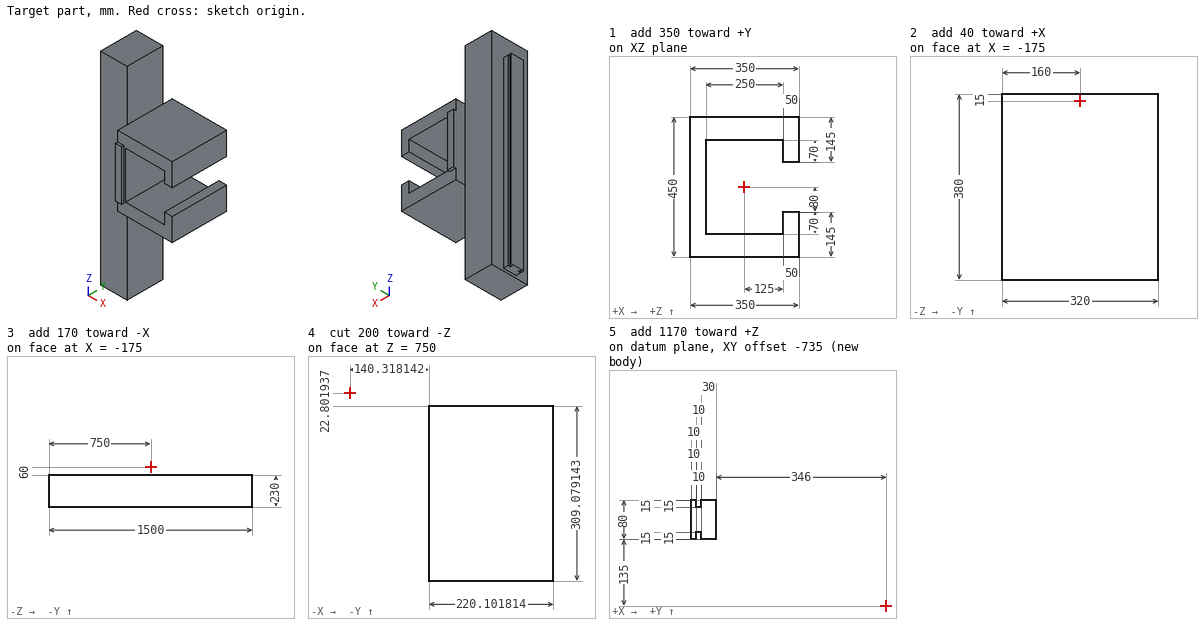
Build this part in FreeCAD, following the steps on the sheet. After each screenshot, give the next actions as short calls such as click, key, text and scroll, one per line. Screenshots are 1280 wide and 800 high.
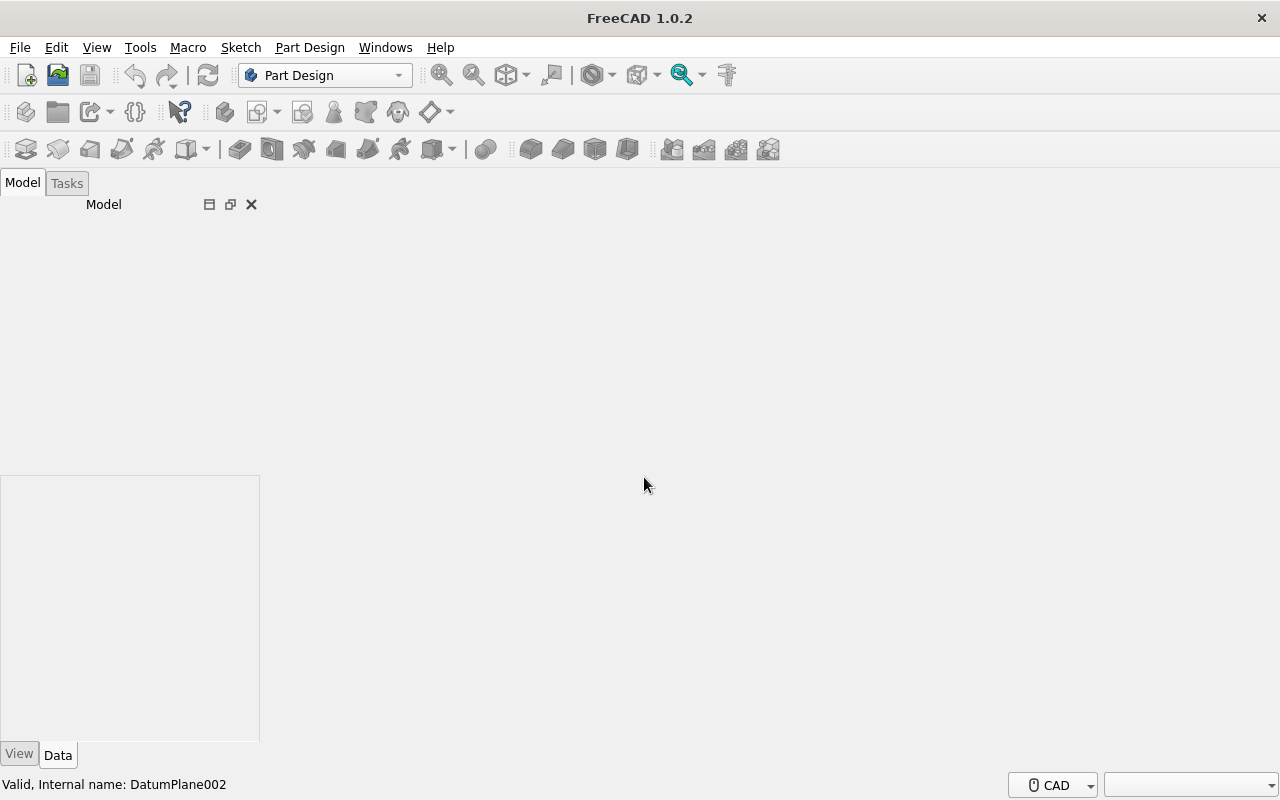
click(26, 76)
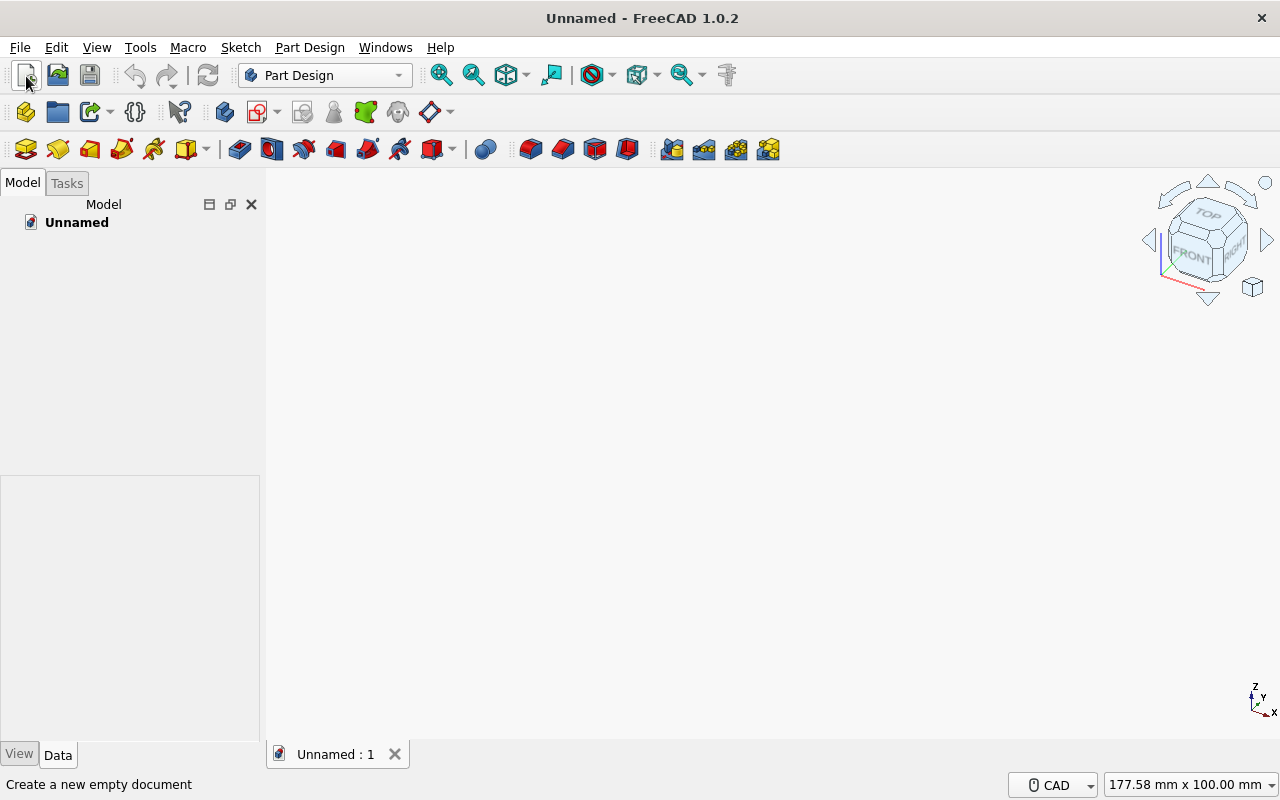
click(258, 112)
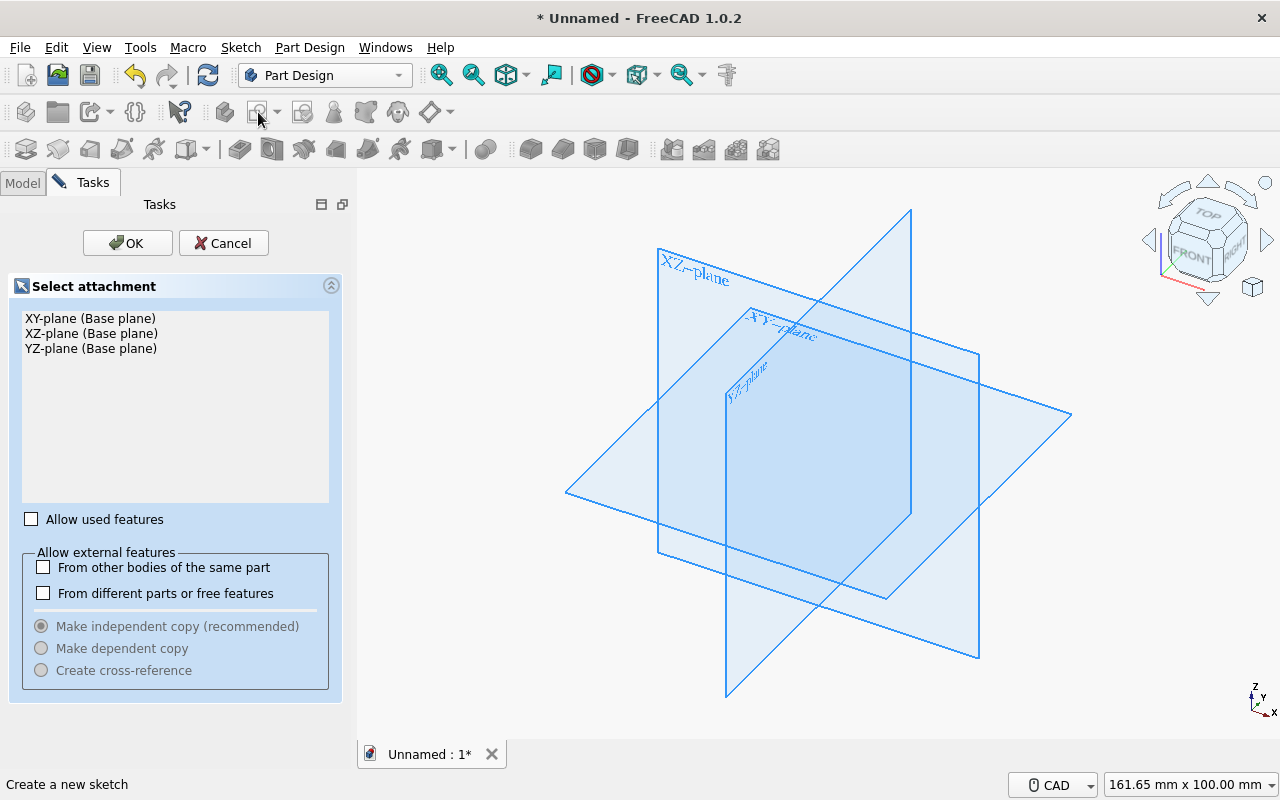
click(82, 334)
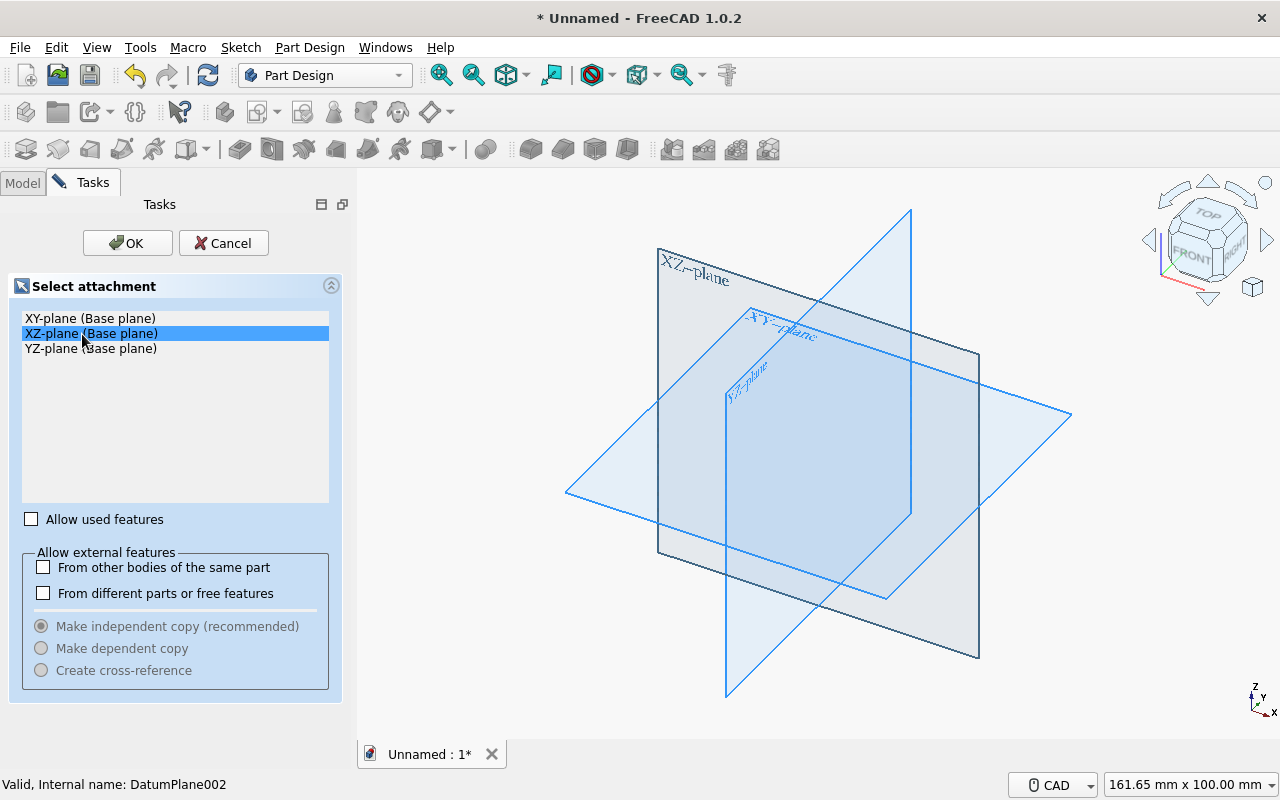
click(128, 243)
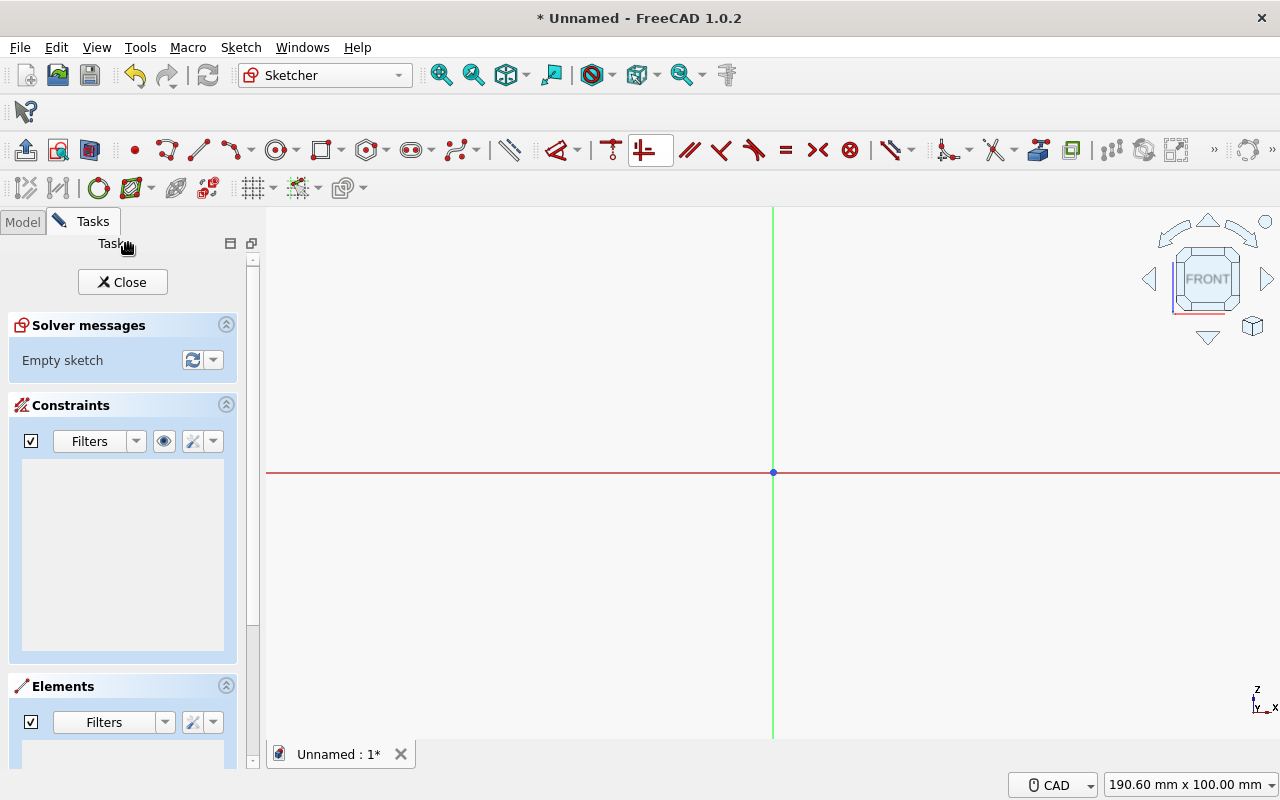
scroll(694, 473, down, 10)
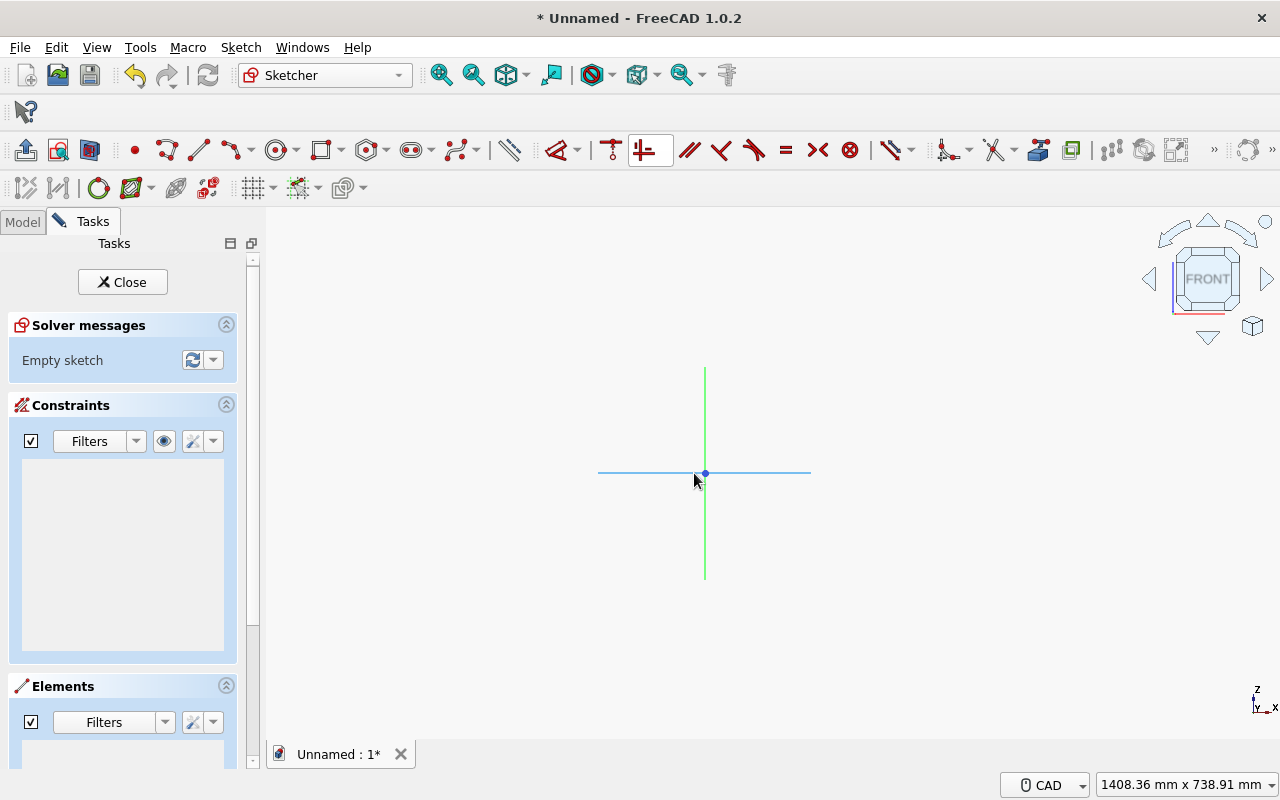
click(168, 150)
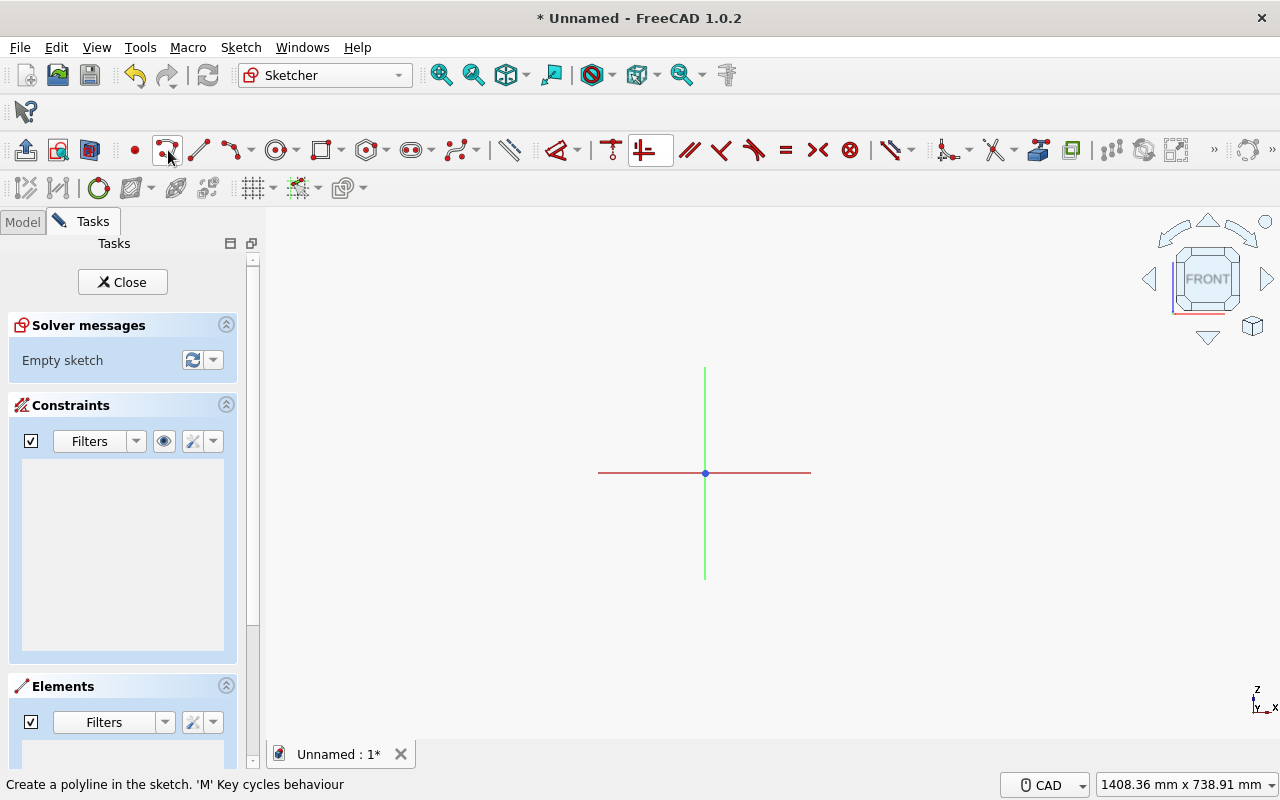
click(795, 531)
click(831, 531)
click(831, 635)
click(579, 635)
click(579, 311)
click(831, 311)
click(831, 416)
click(795, 416)
click(795, 365)
click(615, 365)
click(615, 581)
click(795, 581)
click(795, 532)
key(Escape)
key(Escape)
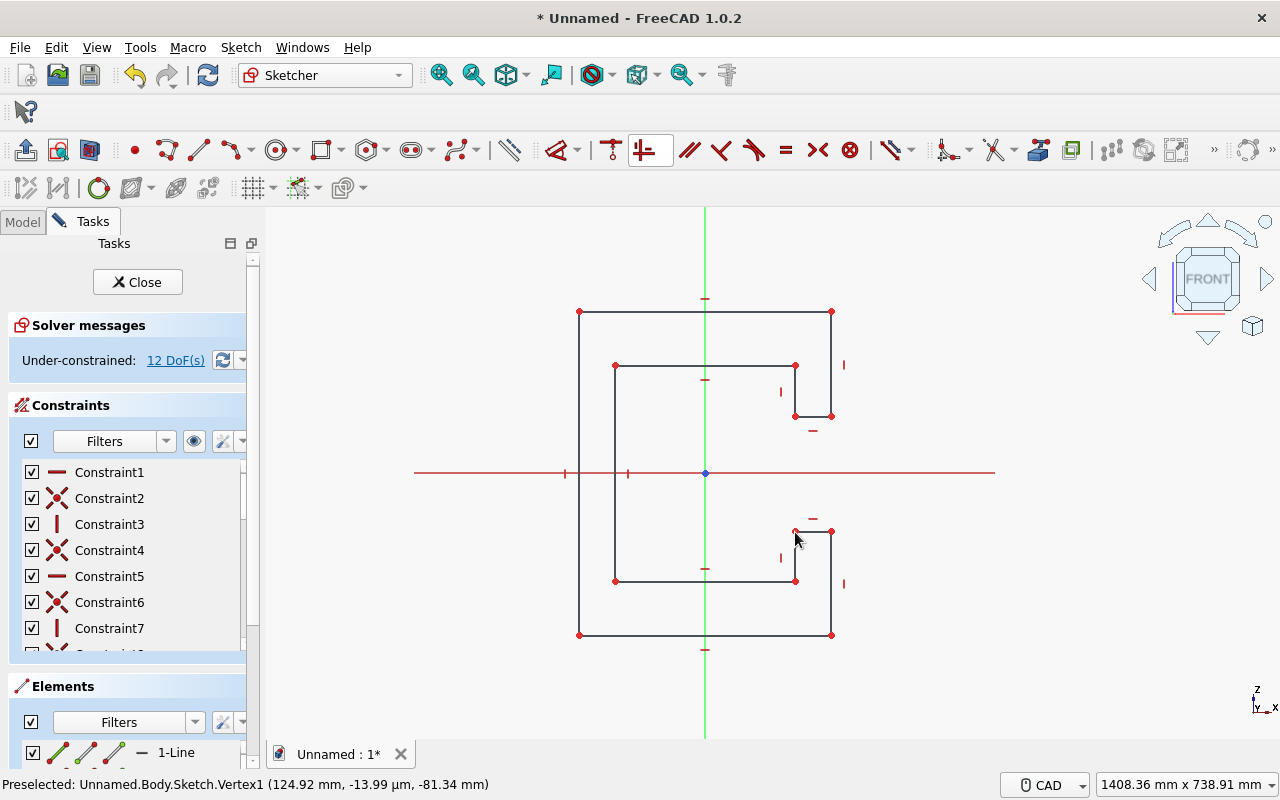
click(556, 150)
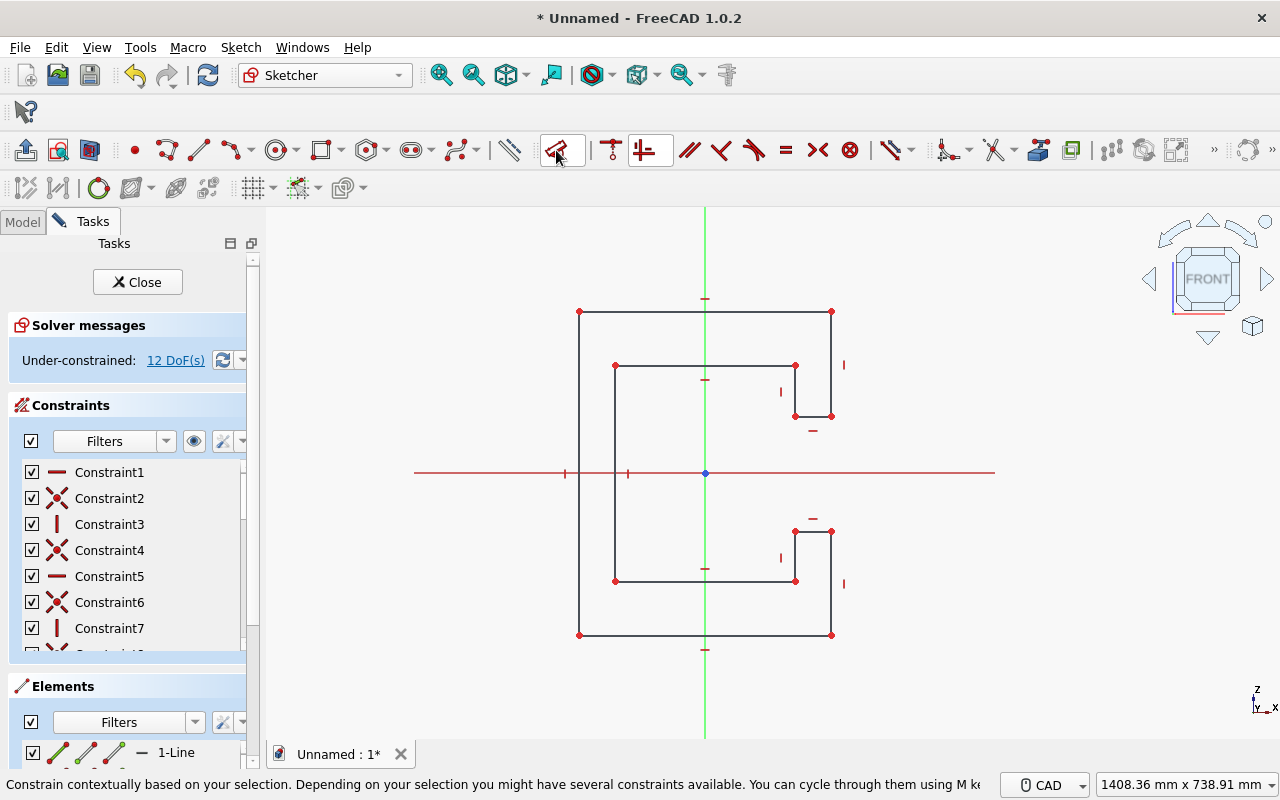
scroll(806, 532, up, 2)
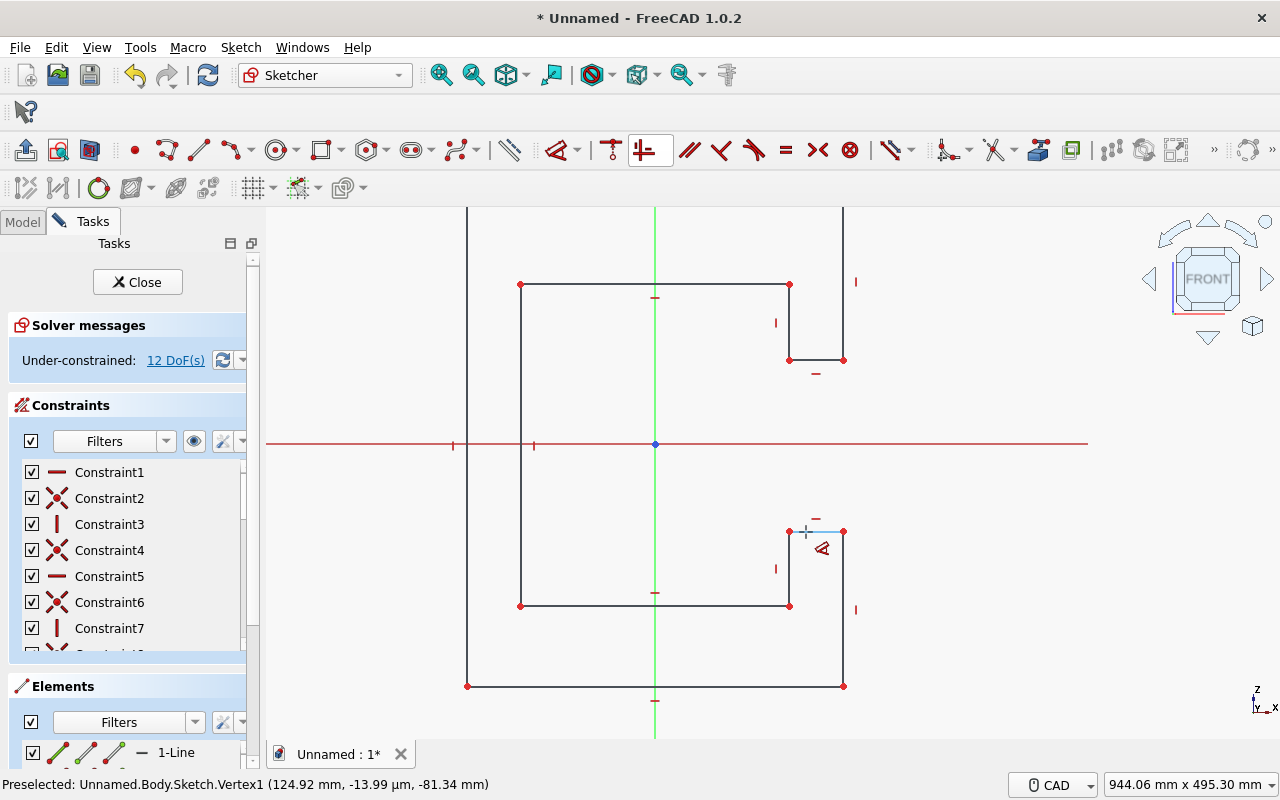
click(805, 532)
click(816, 566)